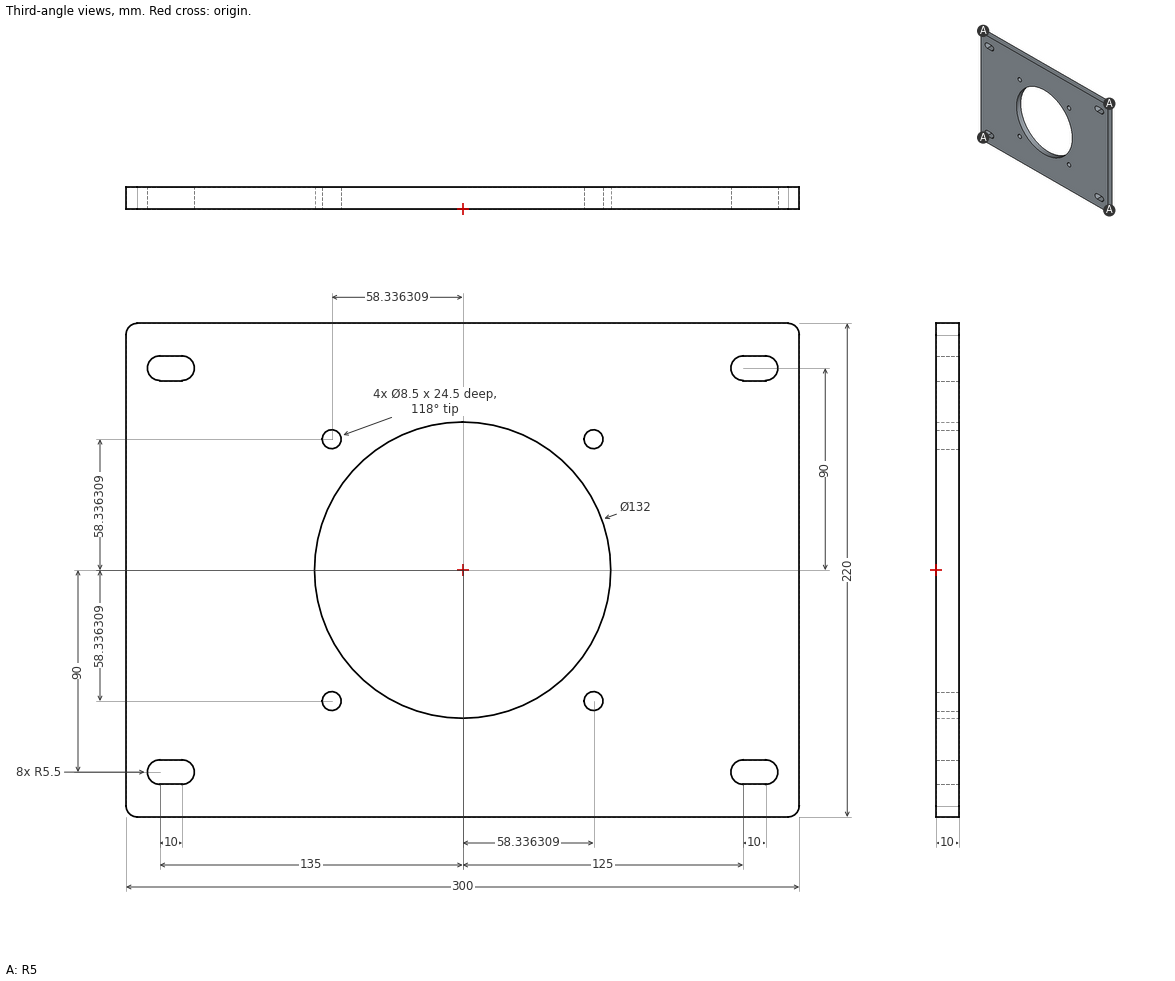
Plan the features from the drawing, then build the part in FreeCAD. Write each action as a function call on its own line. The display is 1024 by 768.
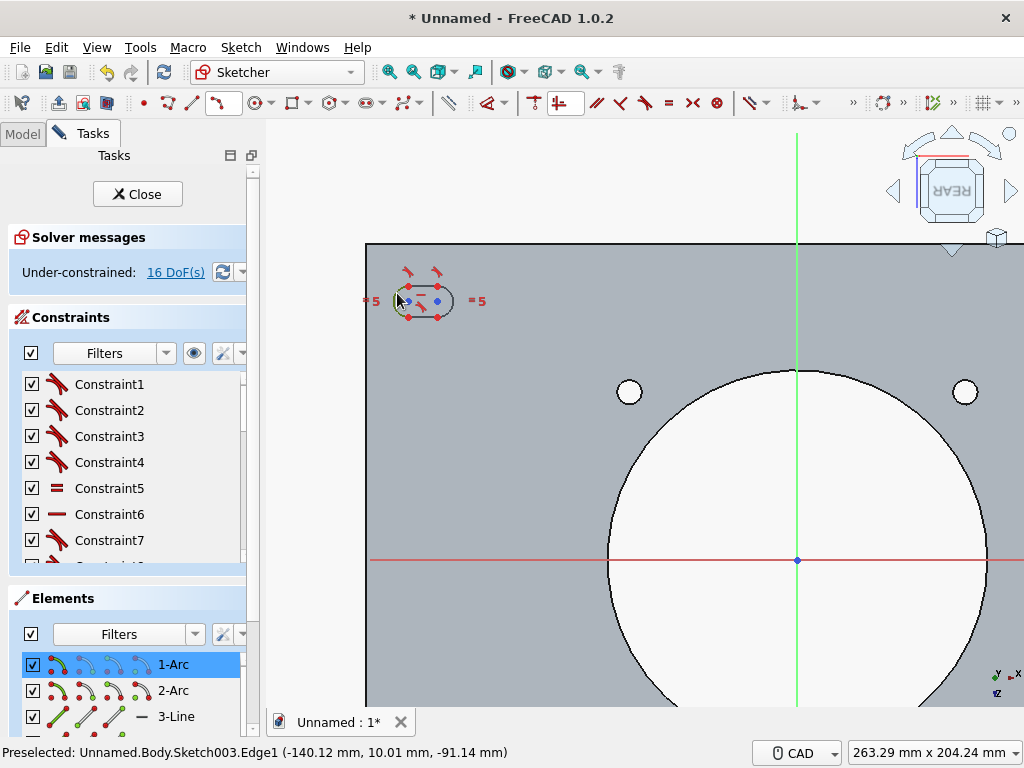
scroll(396, 293, down, 4)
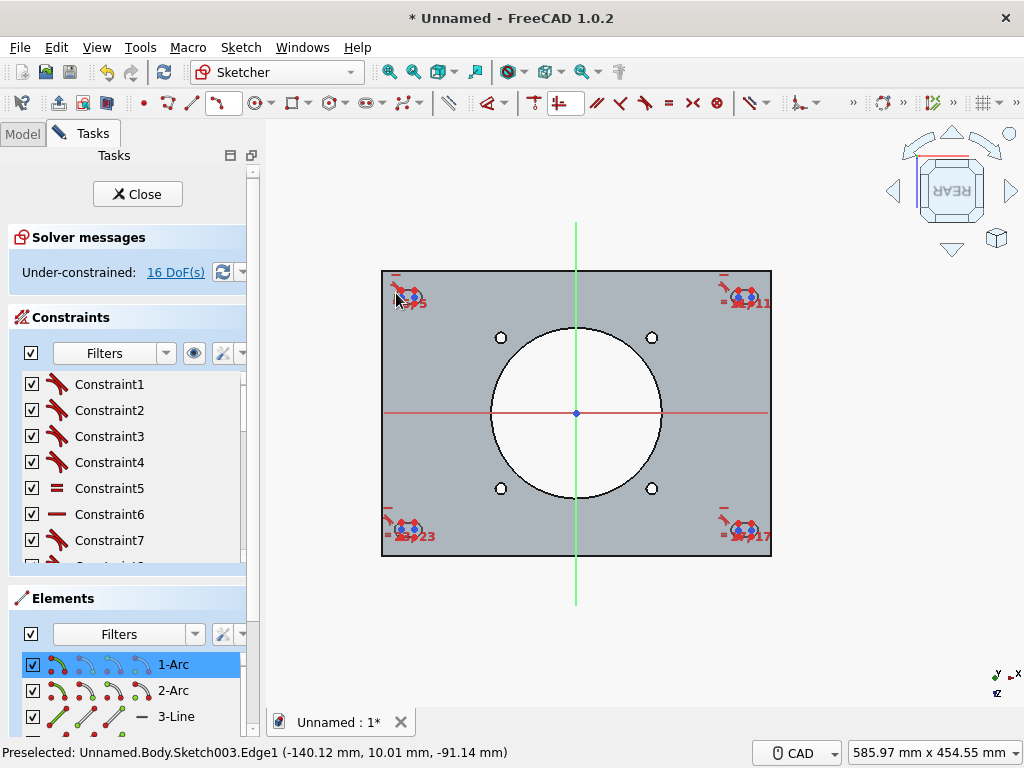
scroll(733, 293, up, 4)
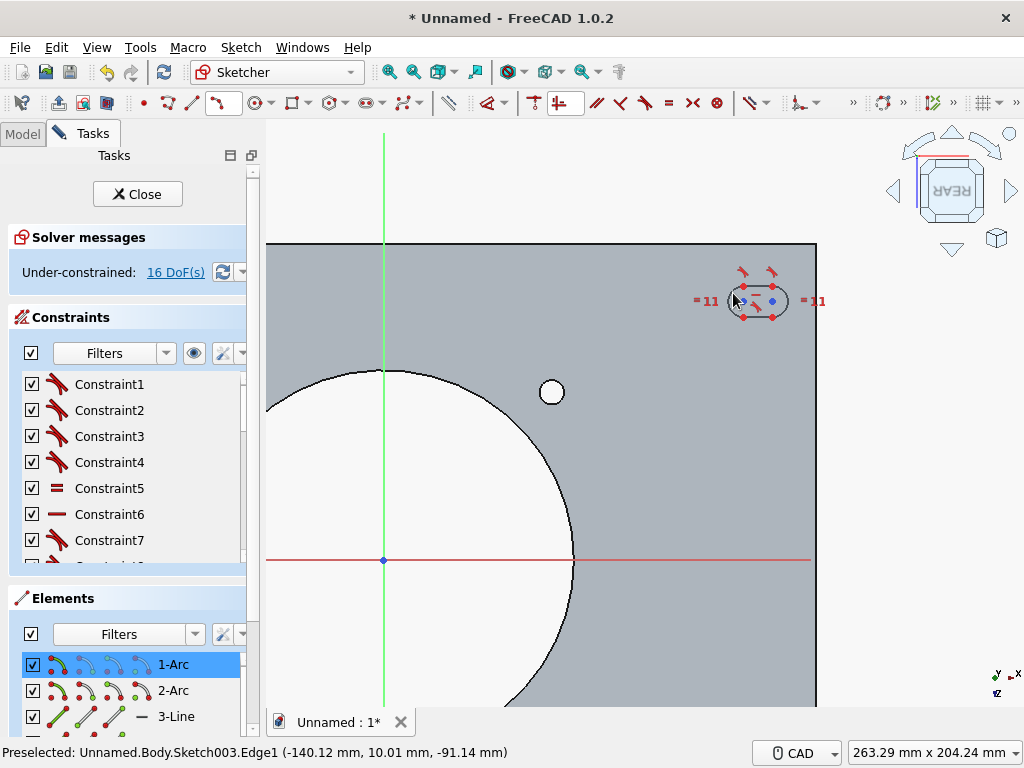
click(731, 293)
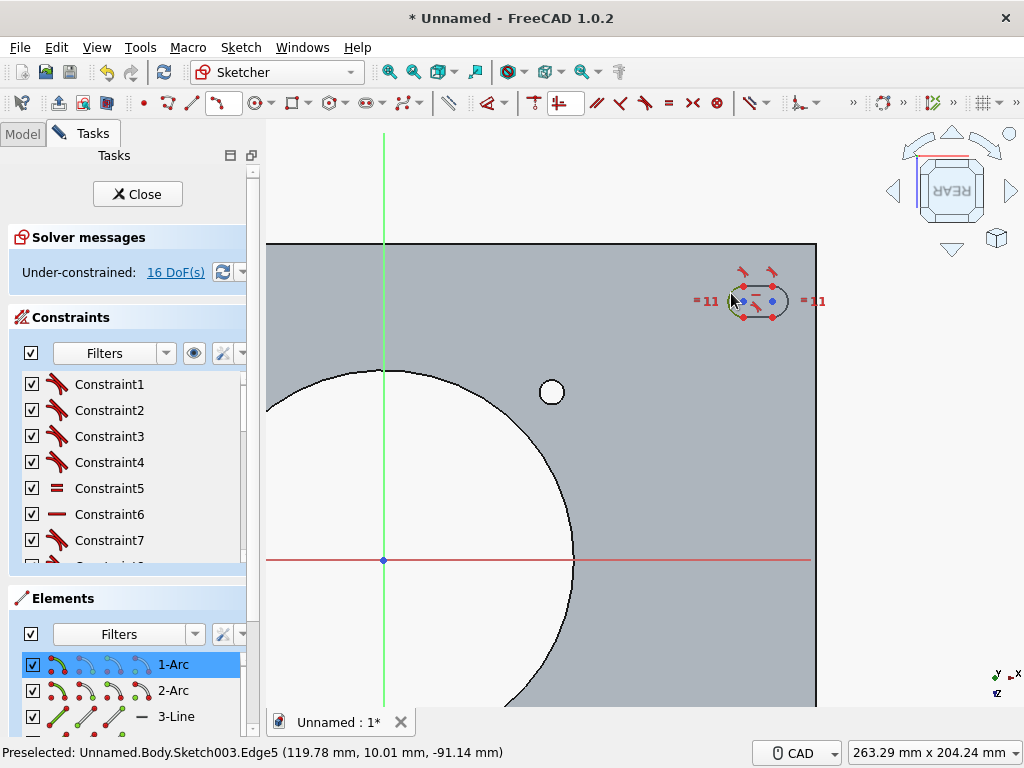
scroll(734, 293, down, 4)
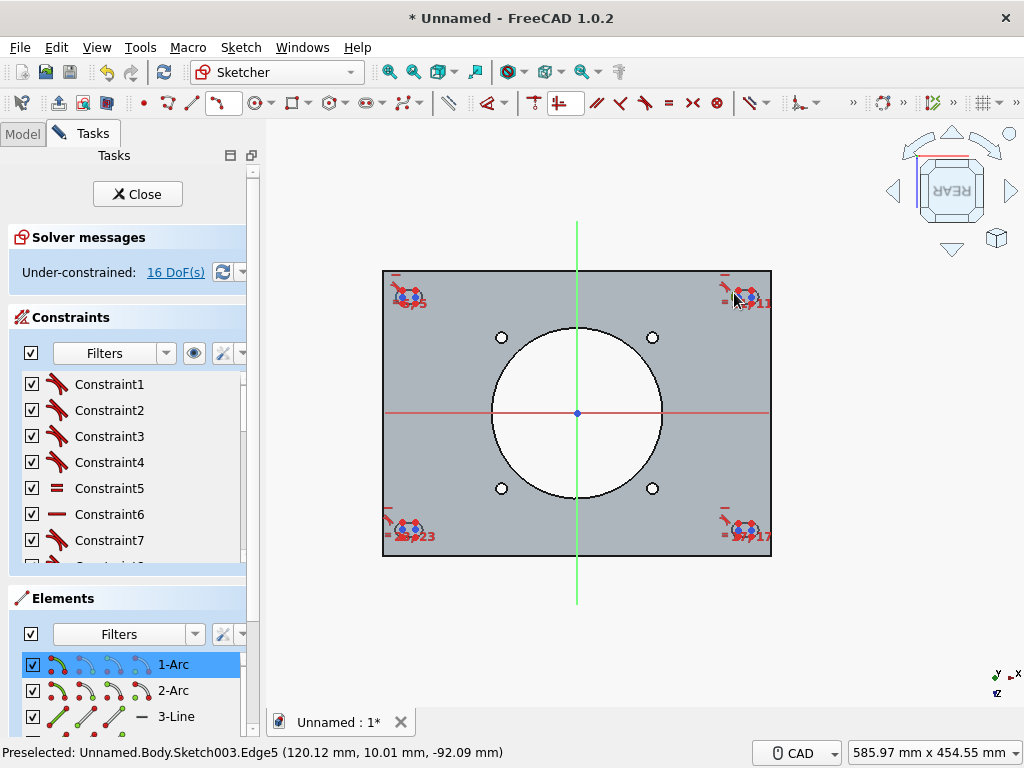
scroll(733, 526, up, 4)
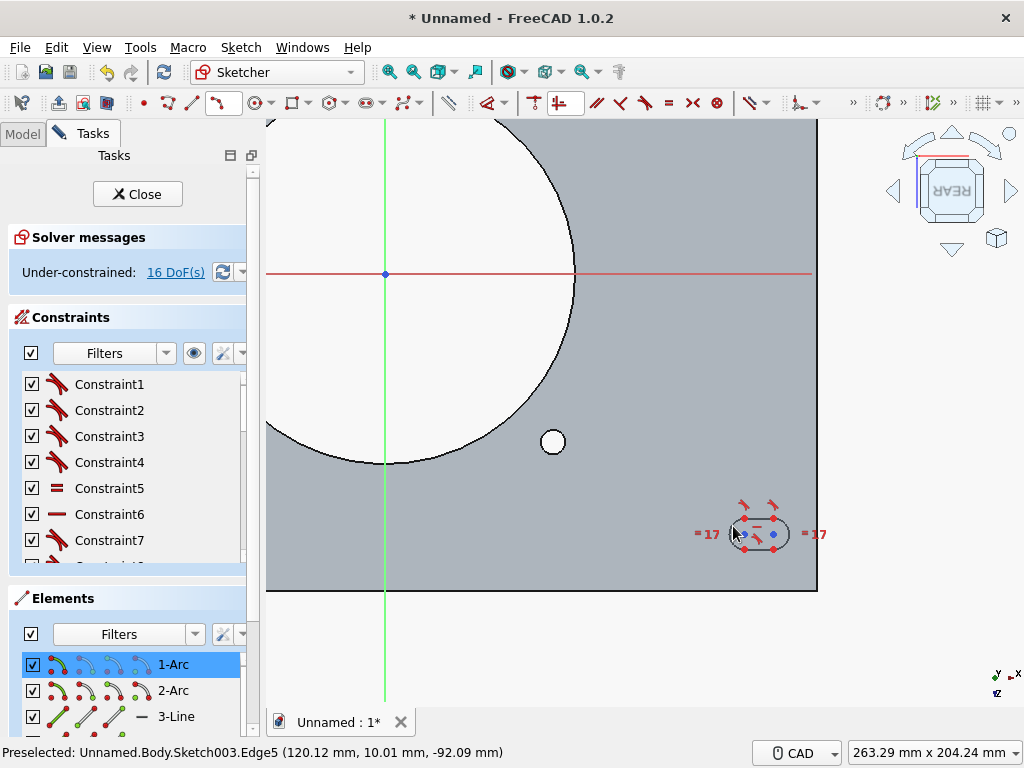
click(732, 525)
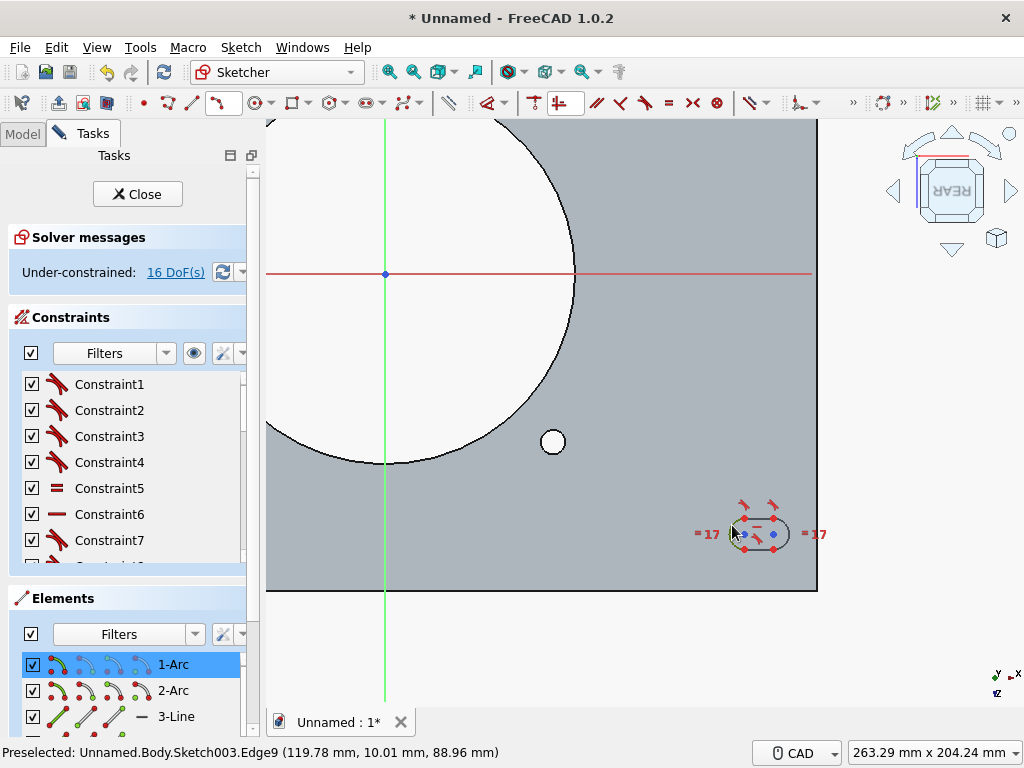
scroll(733, 526, down, 4)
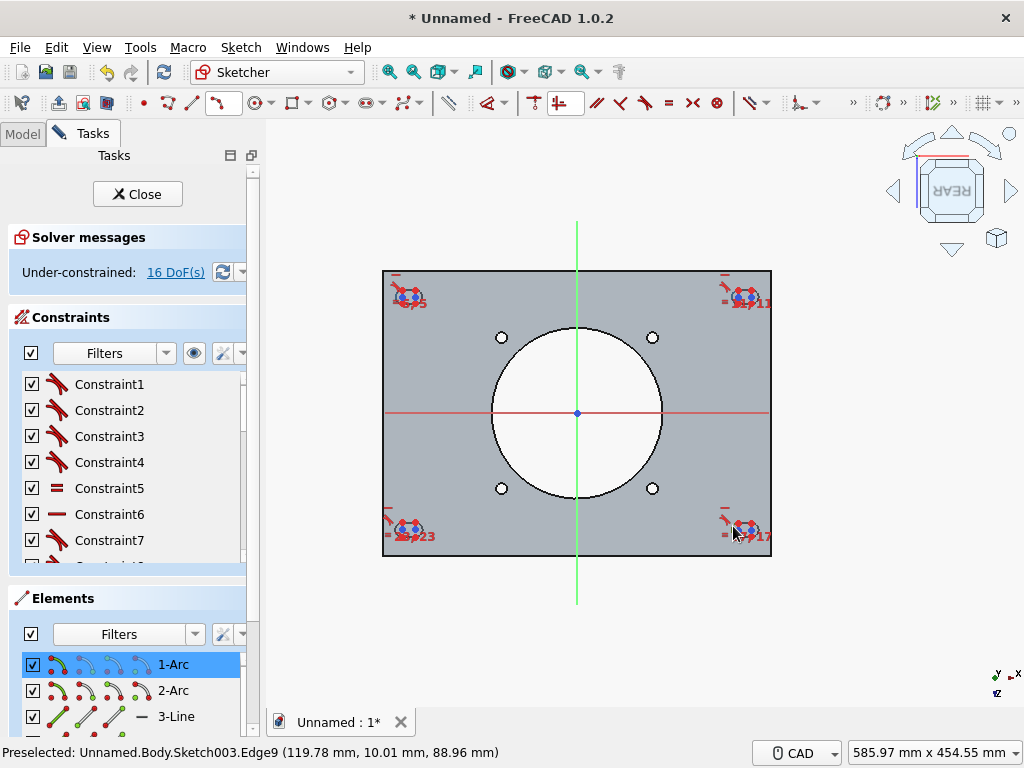
scroll(397, 526, up, 4)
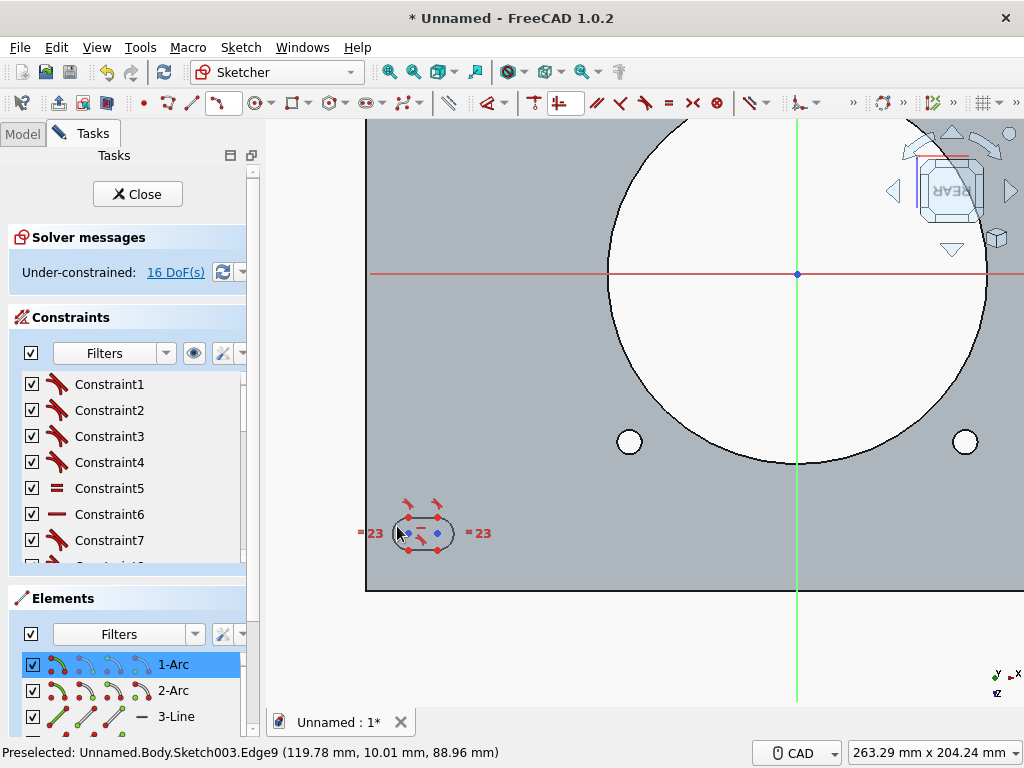
click(396, 524)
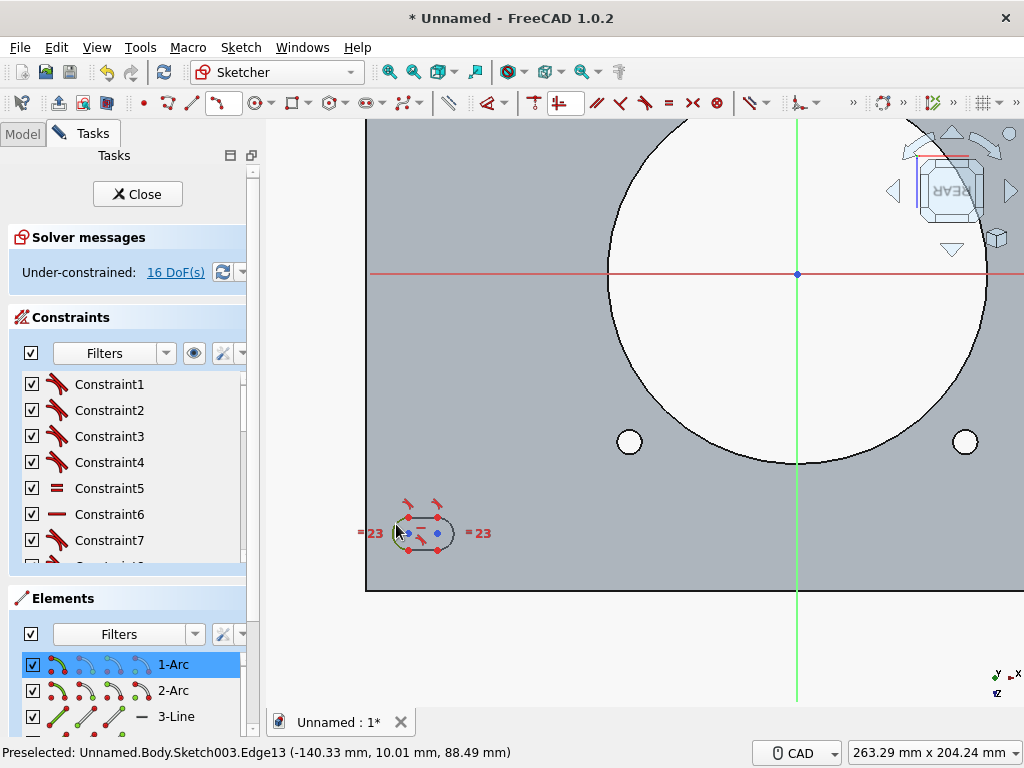
key(e)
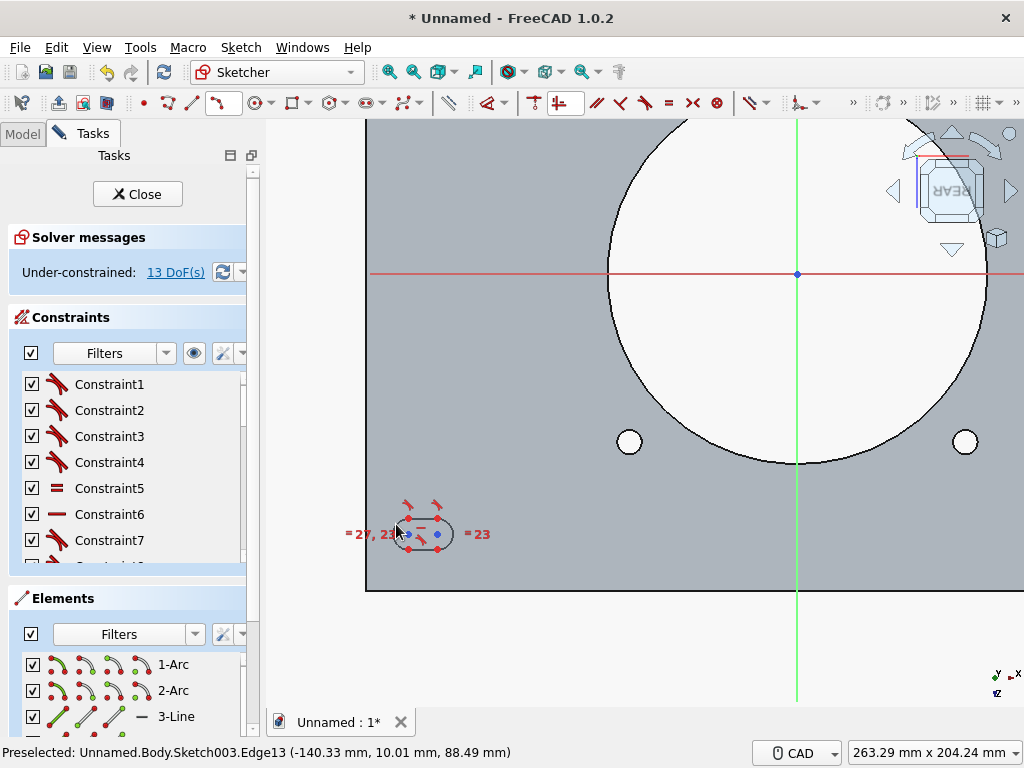
key(d)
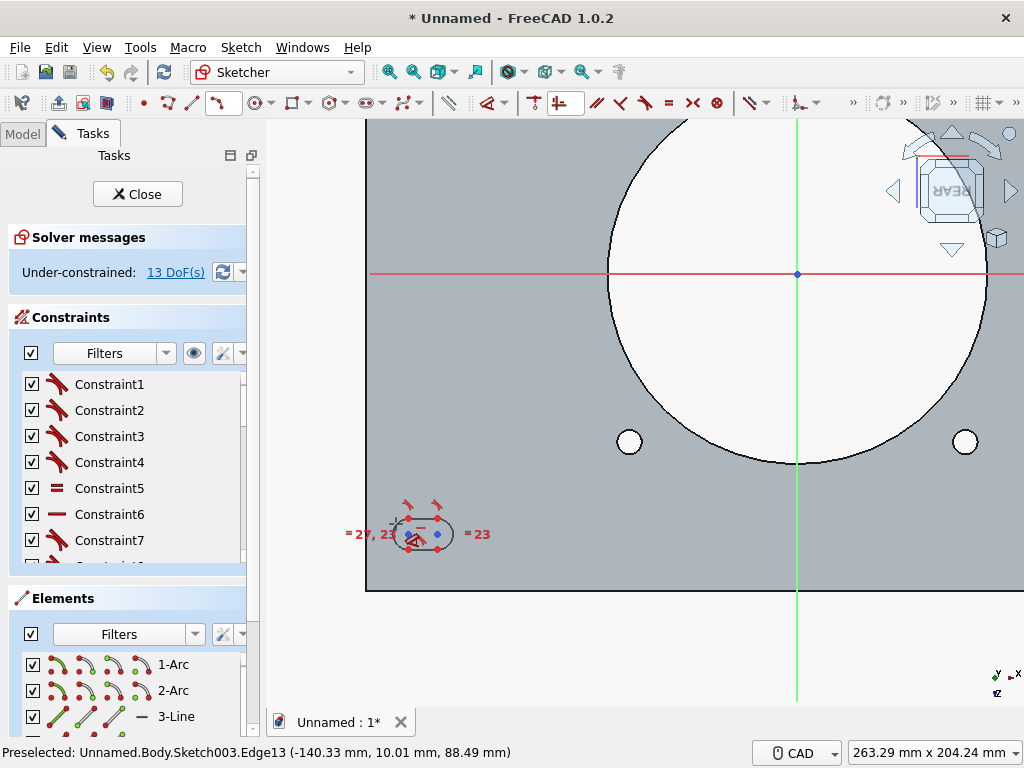
scroll(396, 526, down, 4)